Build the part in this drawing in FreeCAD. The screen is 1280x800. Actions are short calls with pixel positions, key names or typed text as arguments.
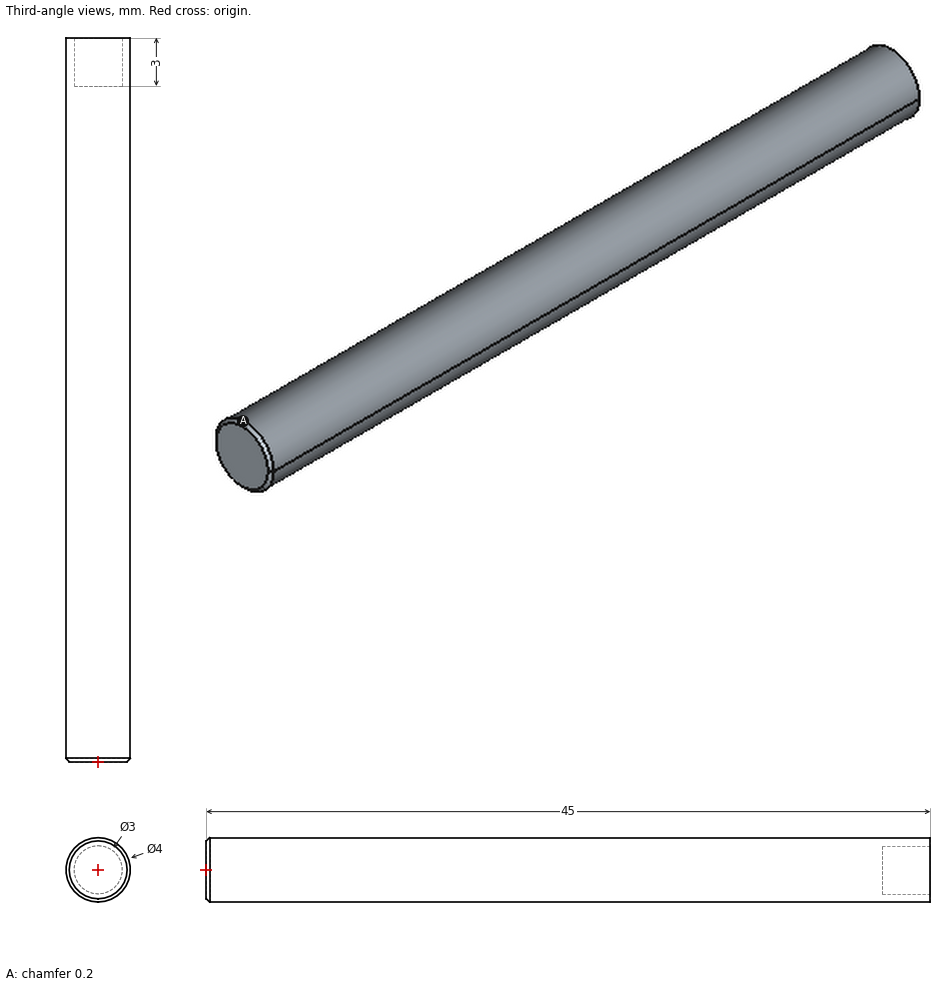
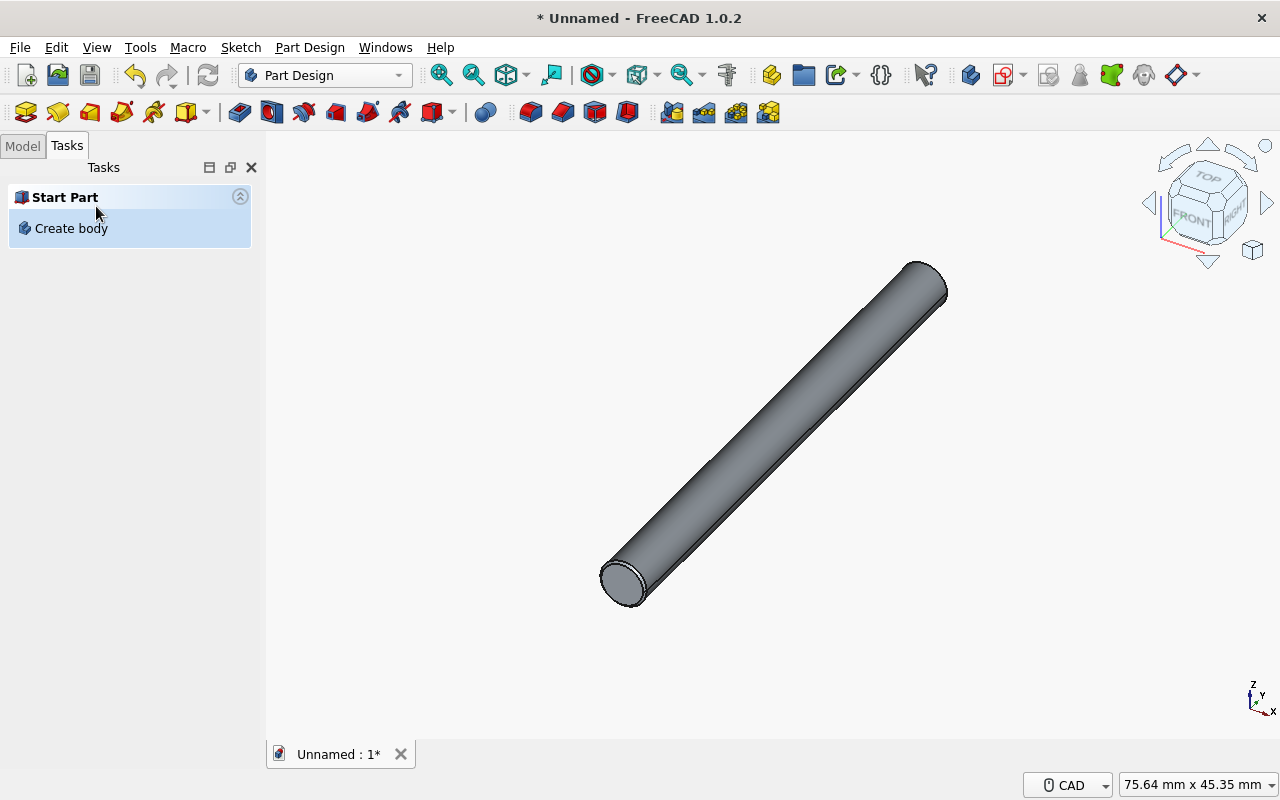
key(4)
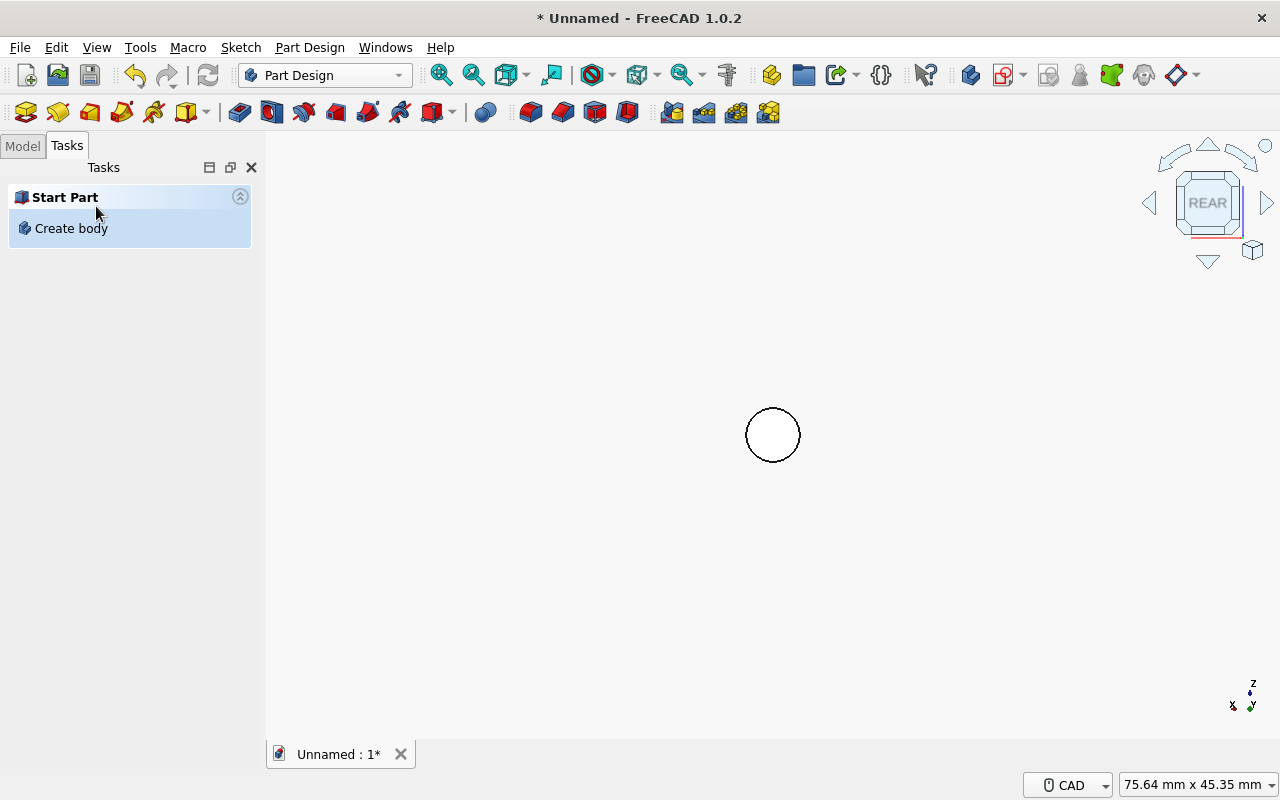
click(442, 76)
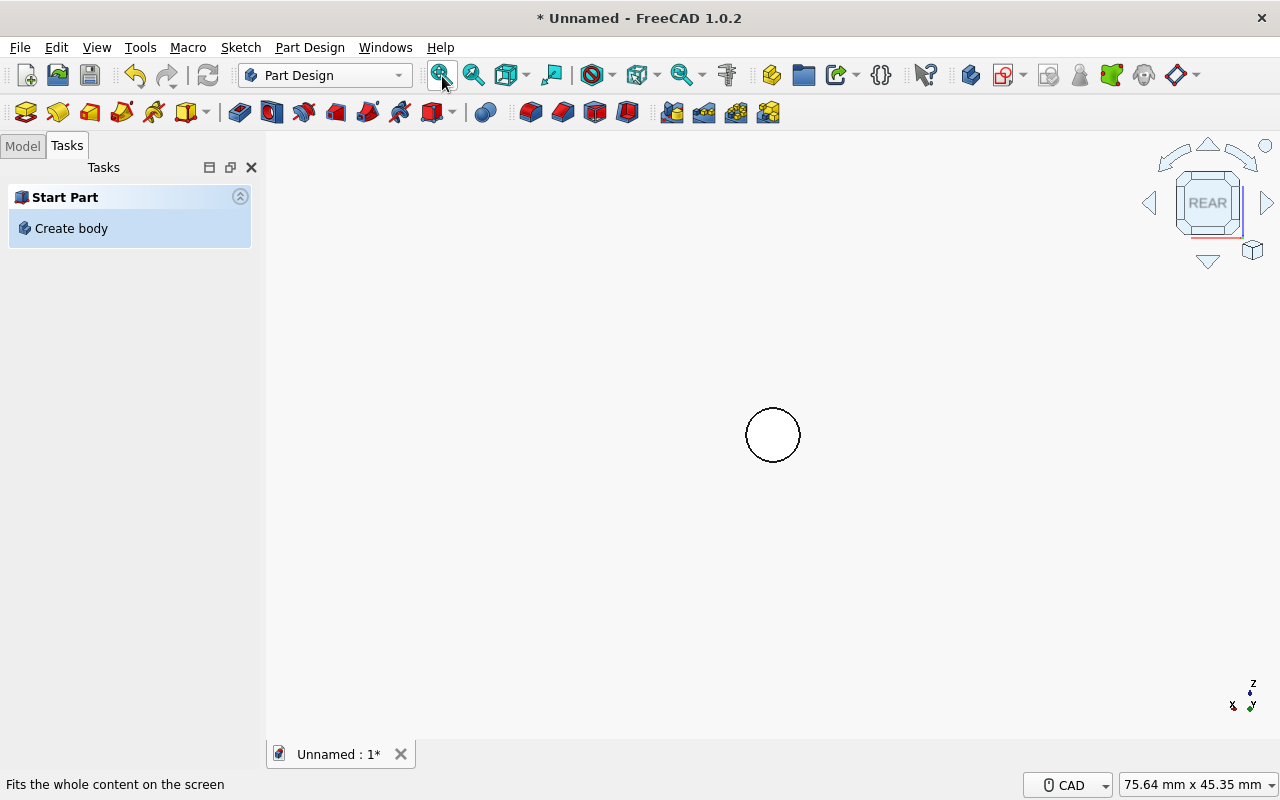
click(773, 434)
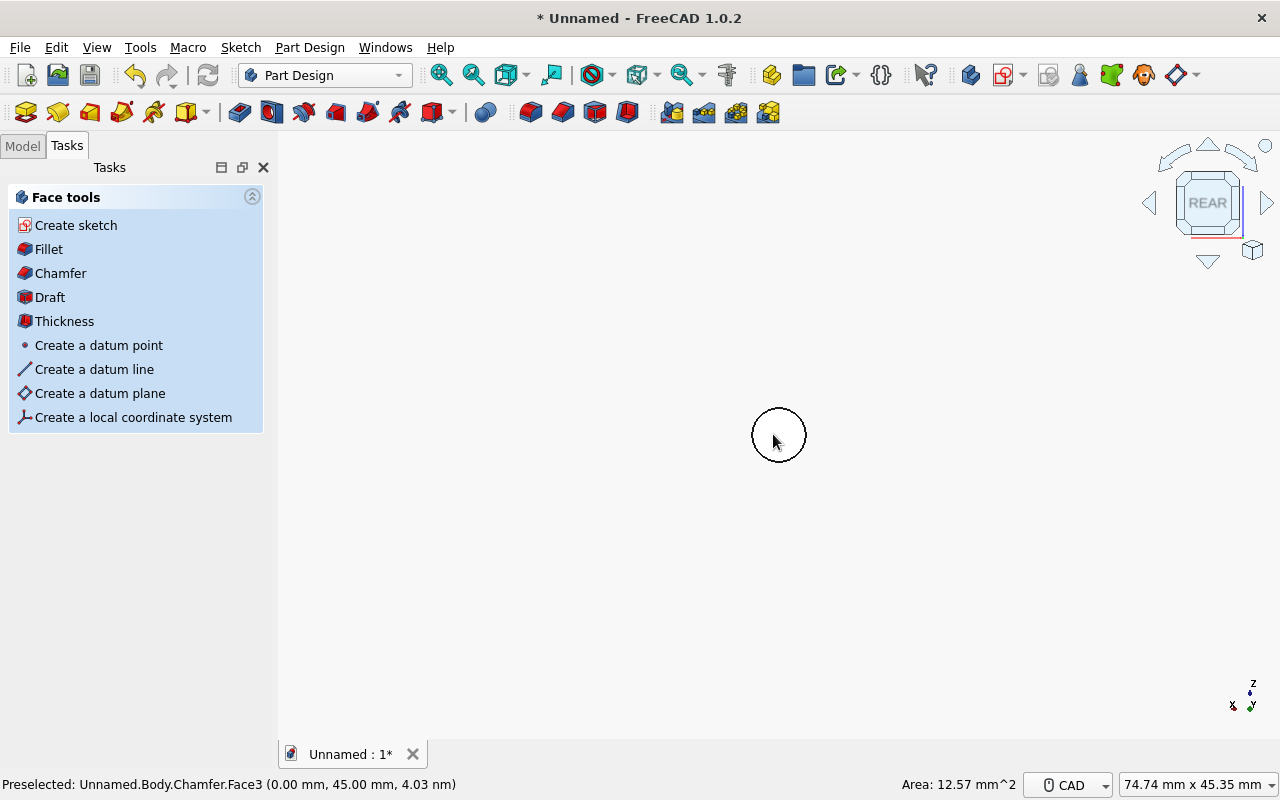
click(1004, 76)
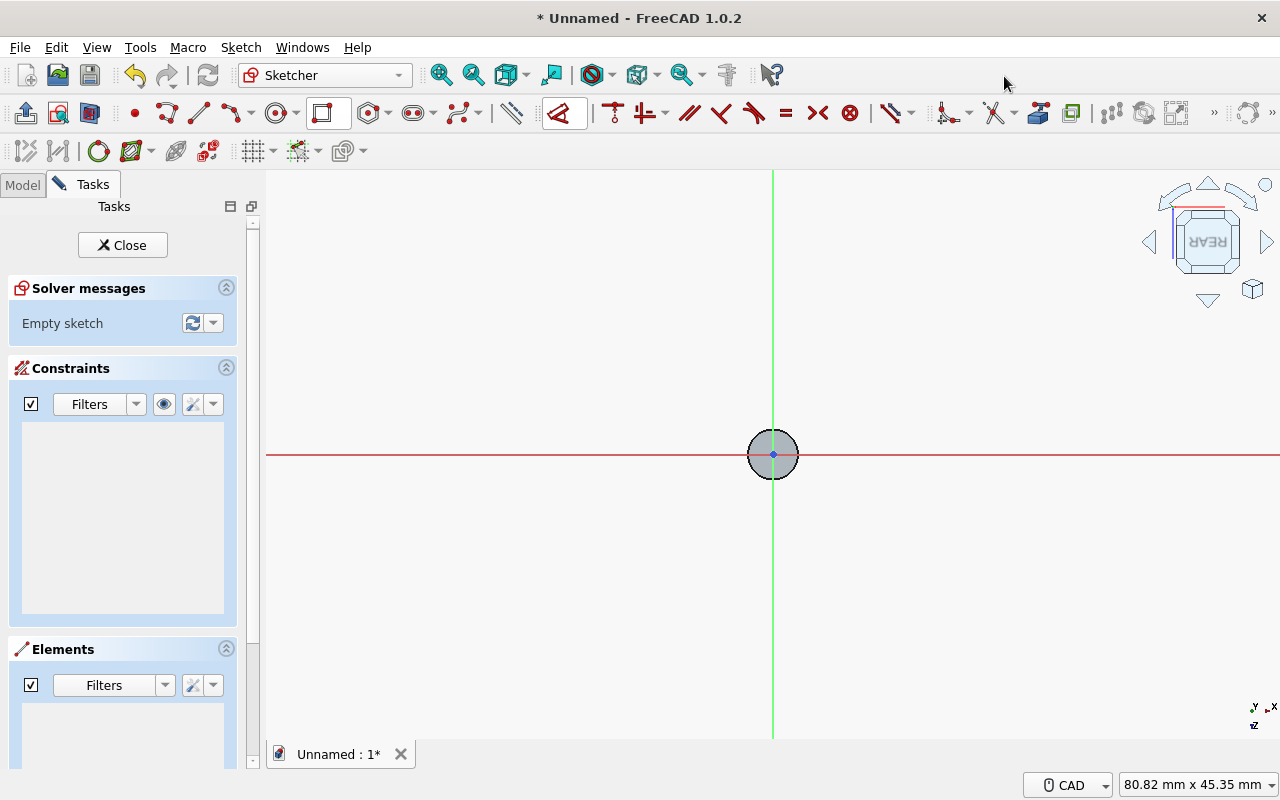
scroll(782, 454, up, 11)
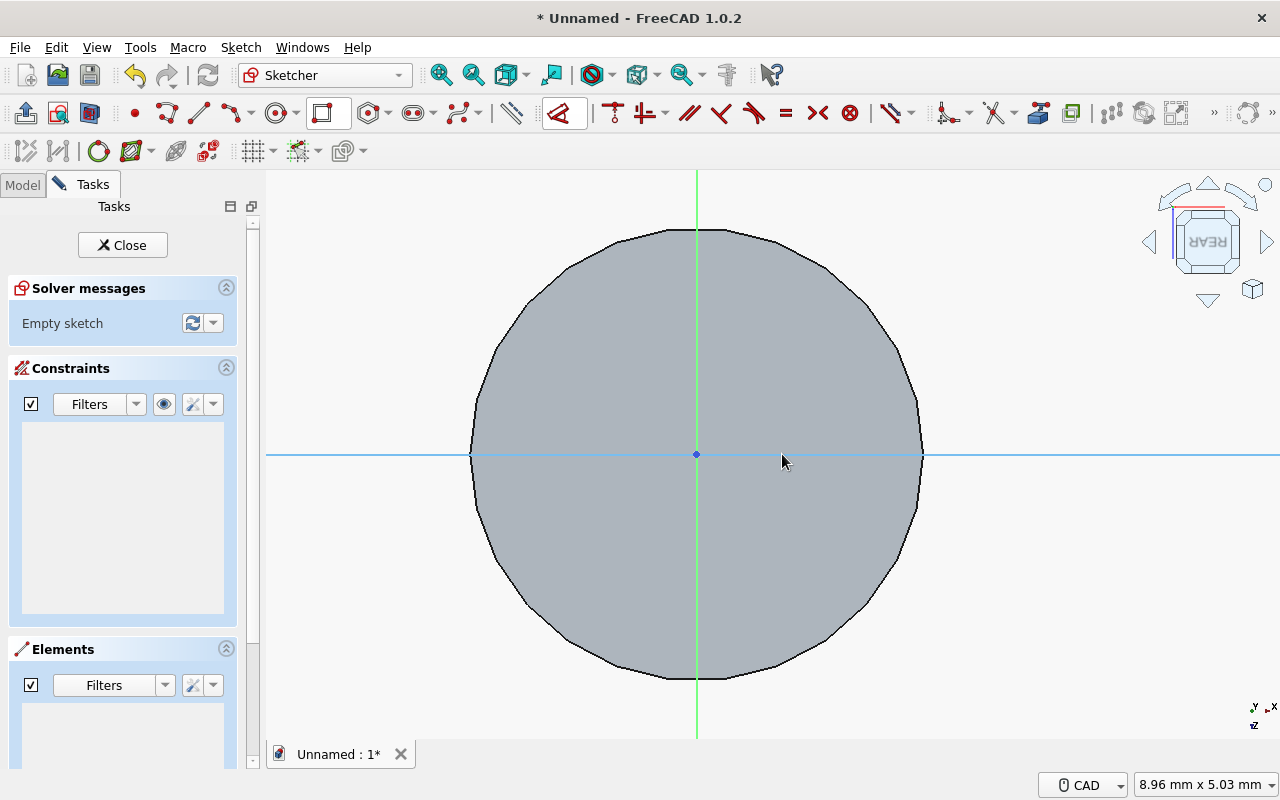
key(g)
key(c)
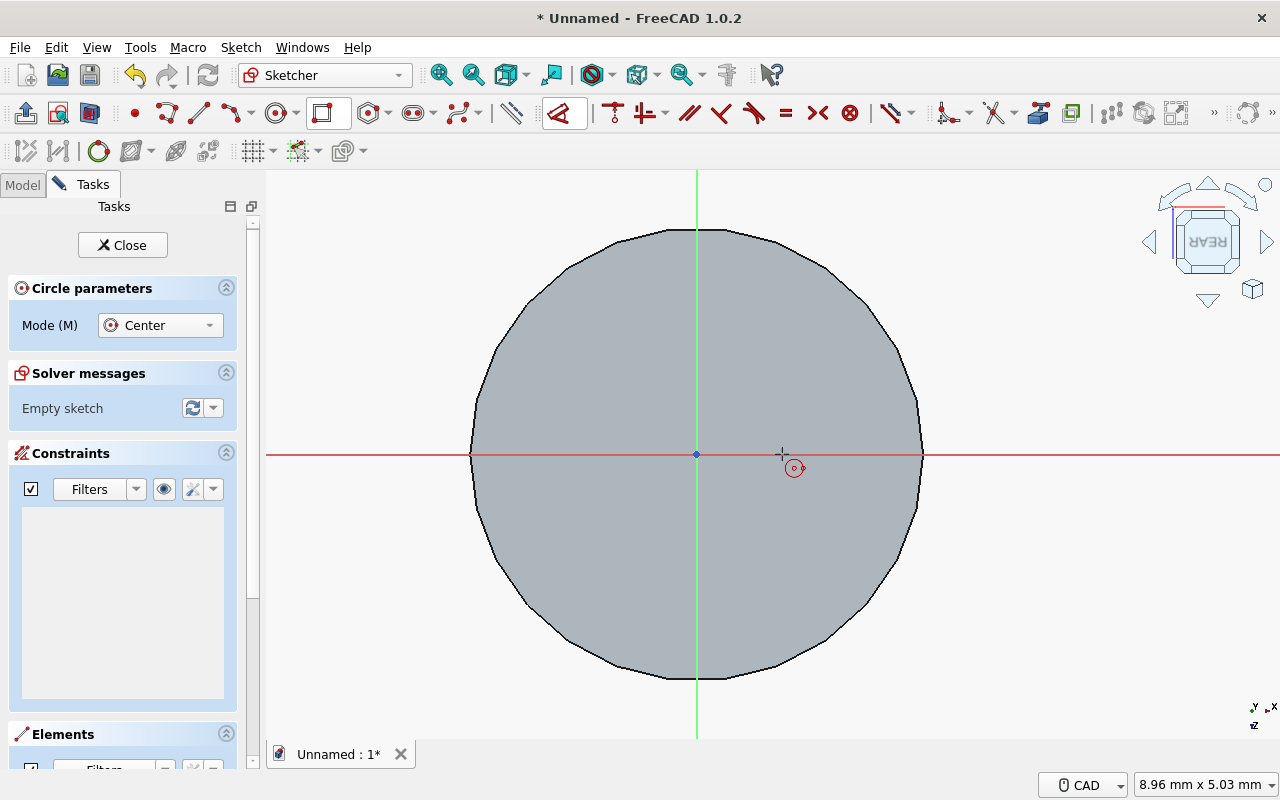
click(697, 454)
click(817, 334)
key(Escape)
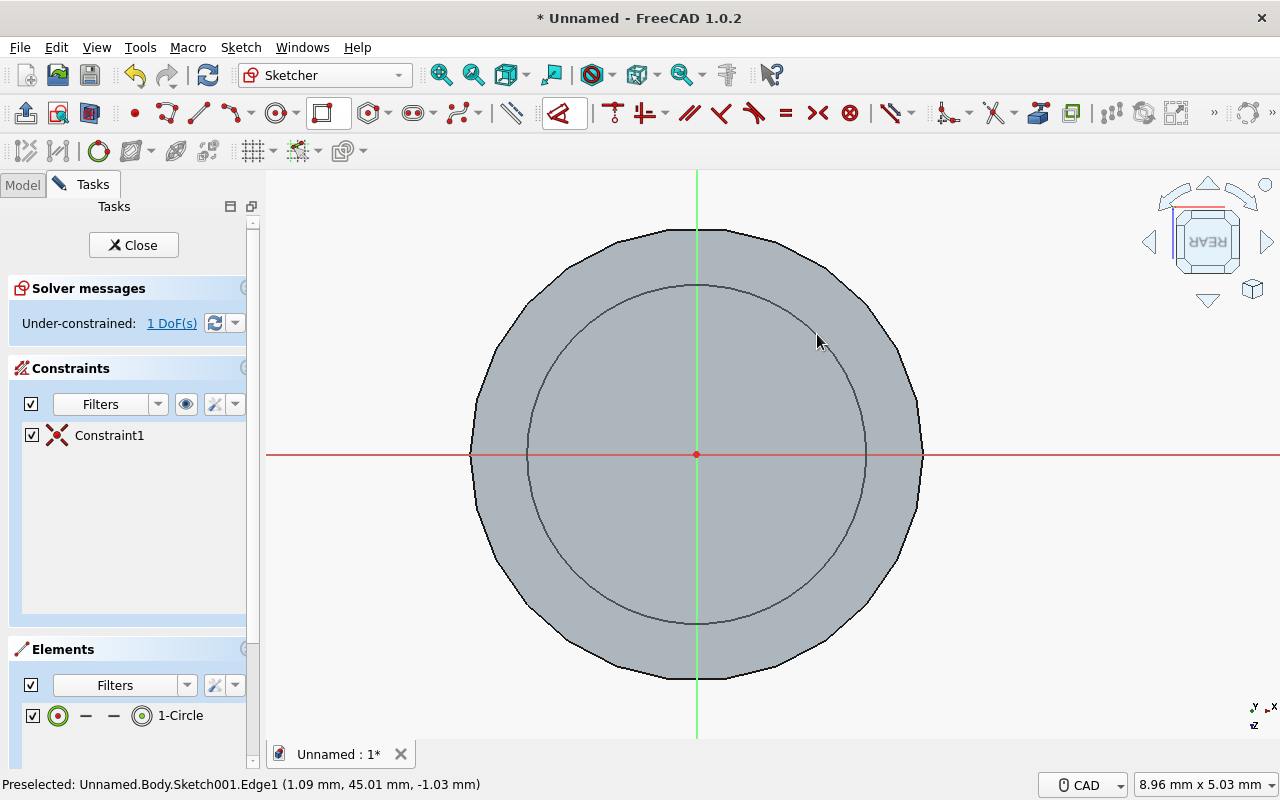
click(558, 114)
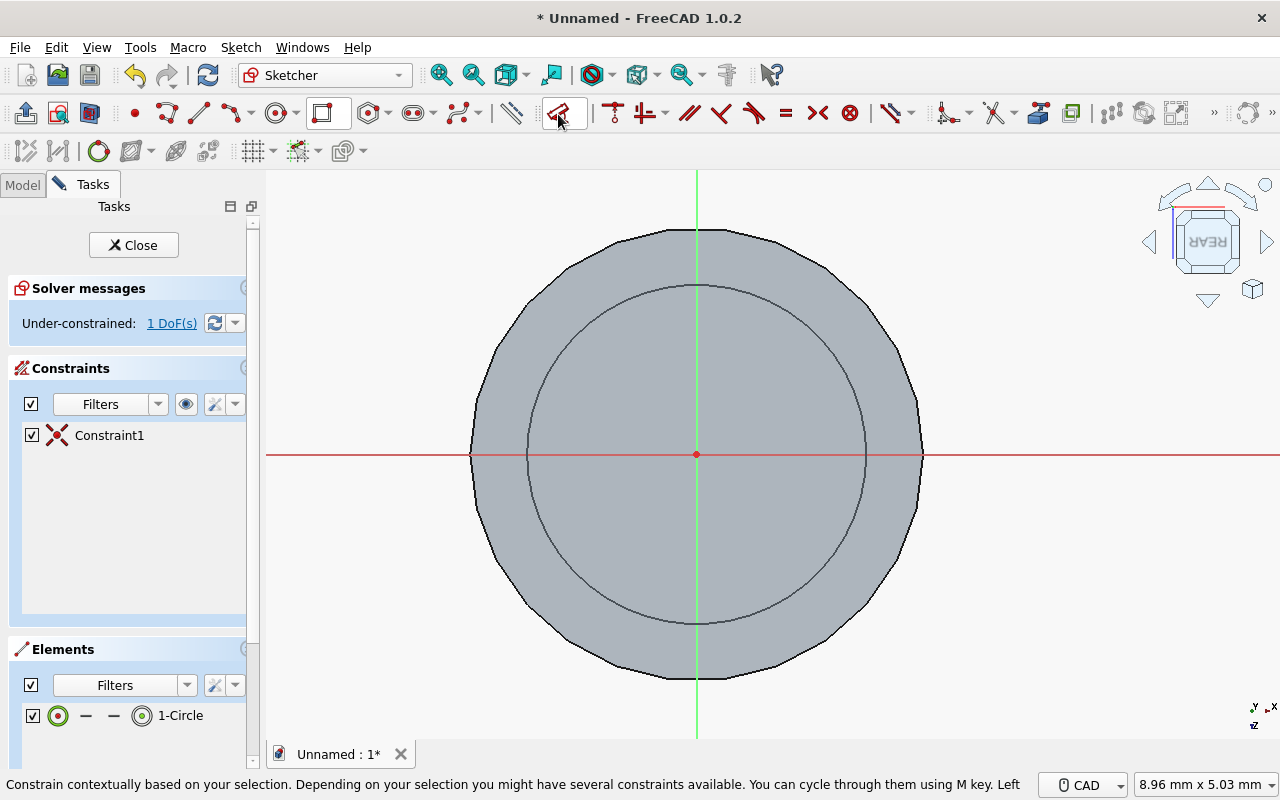
click(816, 334)
click(839, 311)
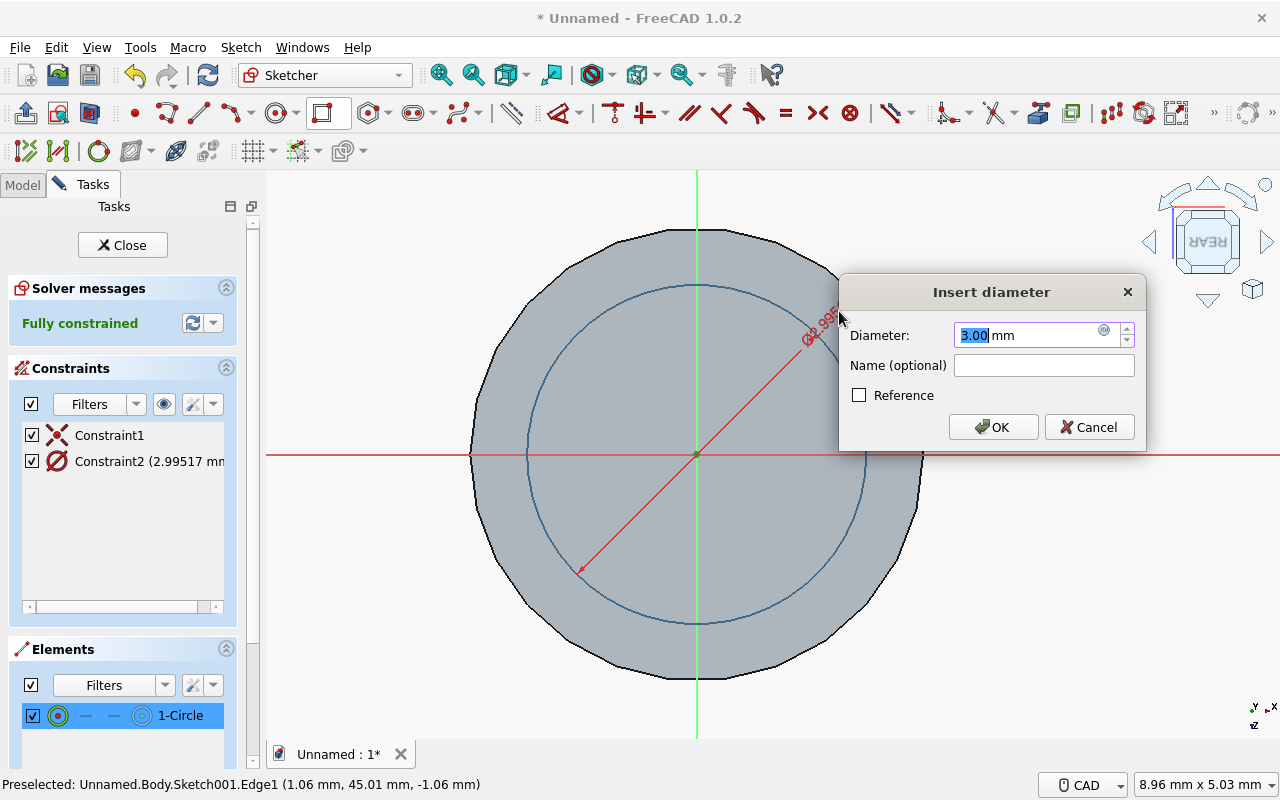
text(3)
key(Return)
key(Escape)